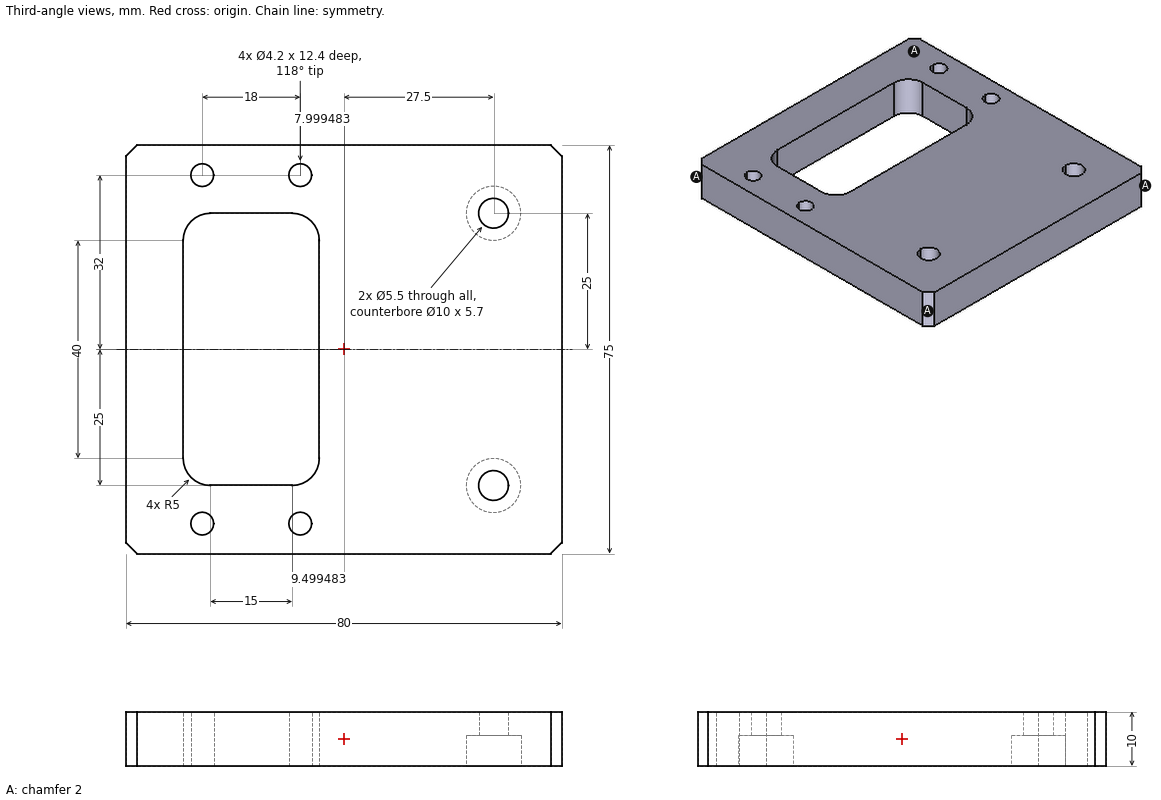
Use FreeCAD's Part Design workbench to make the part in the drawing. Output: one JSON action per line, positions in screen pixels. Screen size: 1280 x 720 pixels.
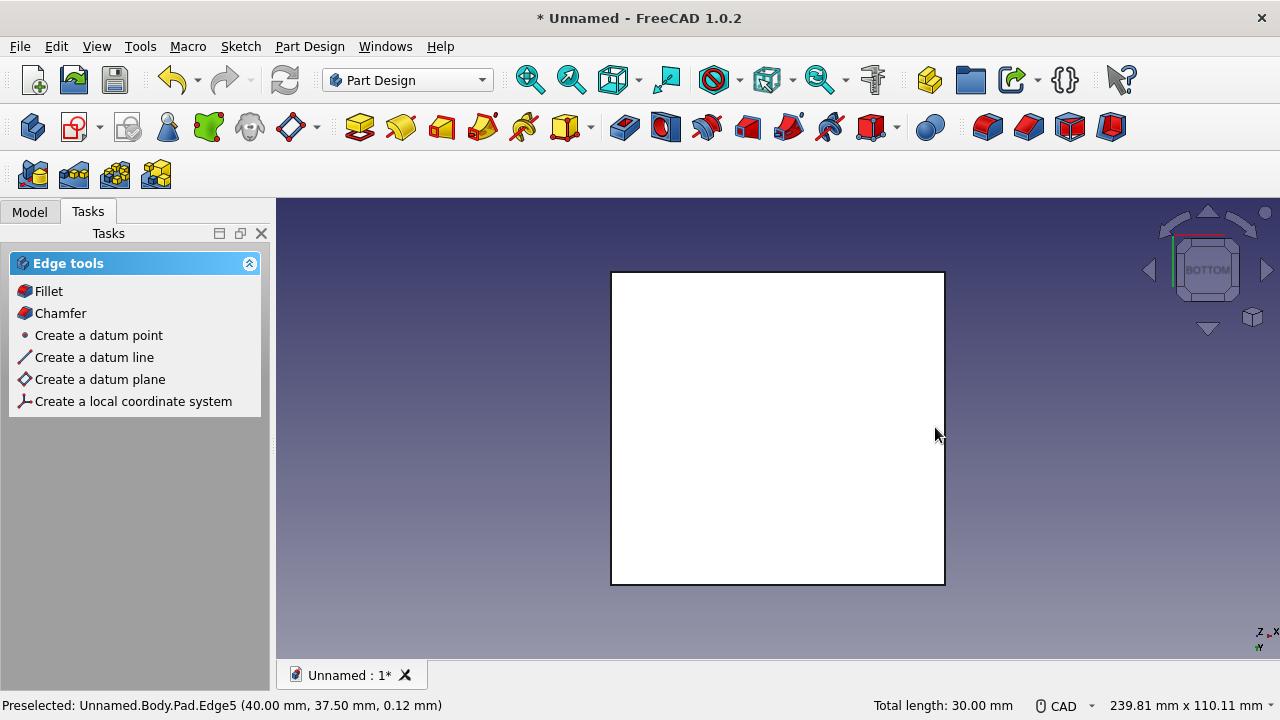
{"action": "key", "text": "4"}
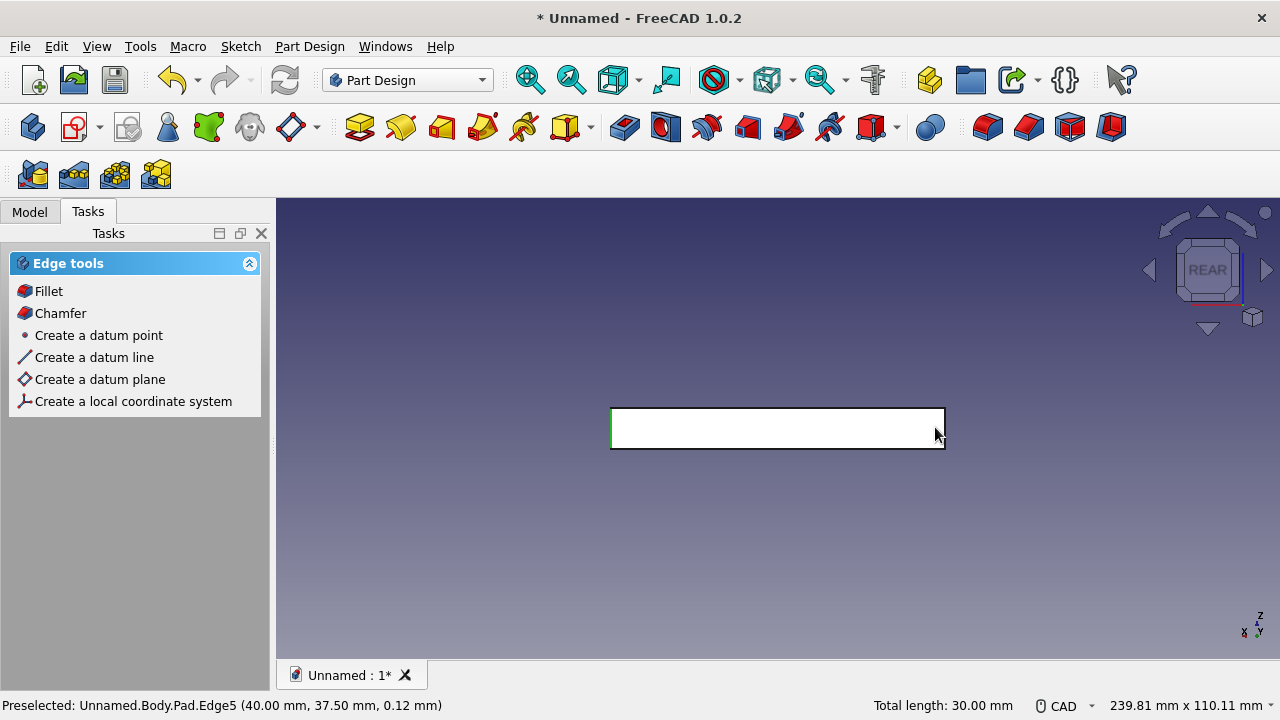
{"action": "key", "text": "v f"}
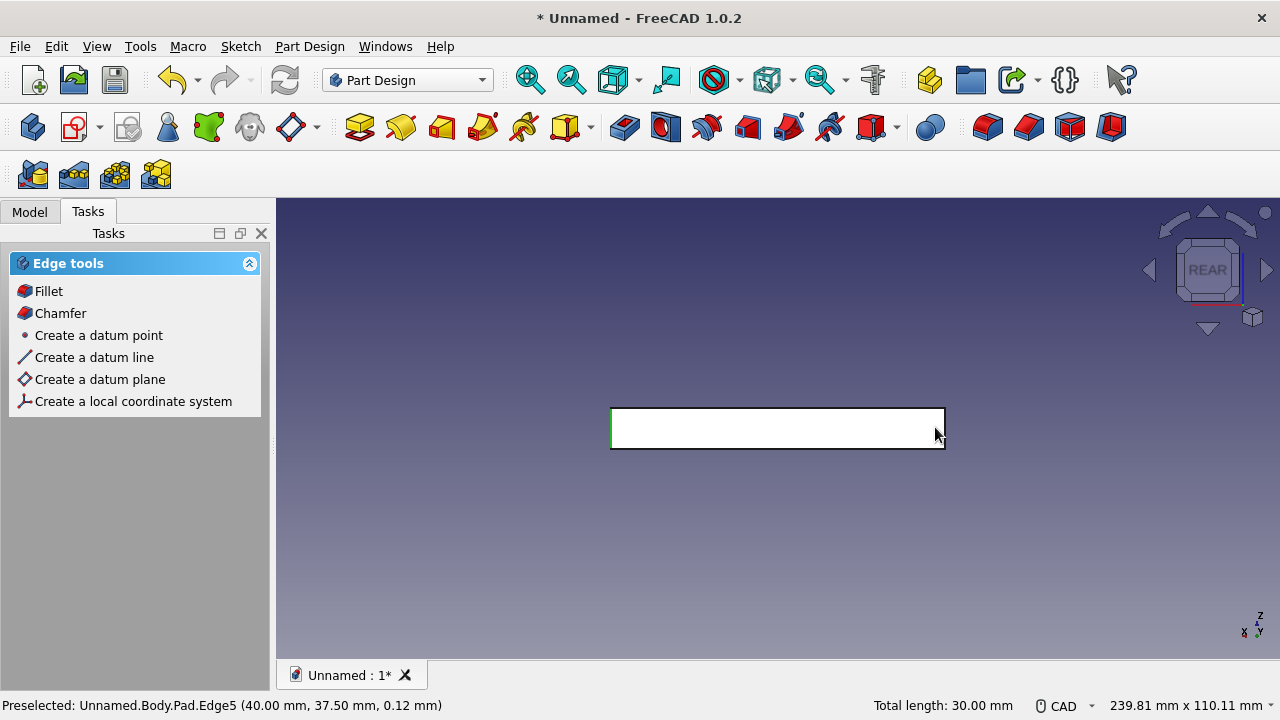
{"action": "left_click", "coordinate": [945, 428], "text": "ctrl"}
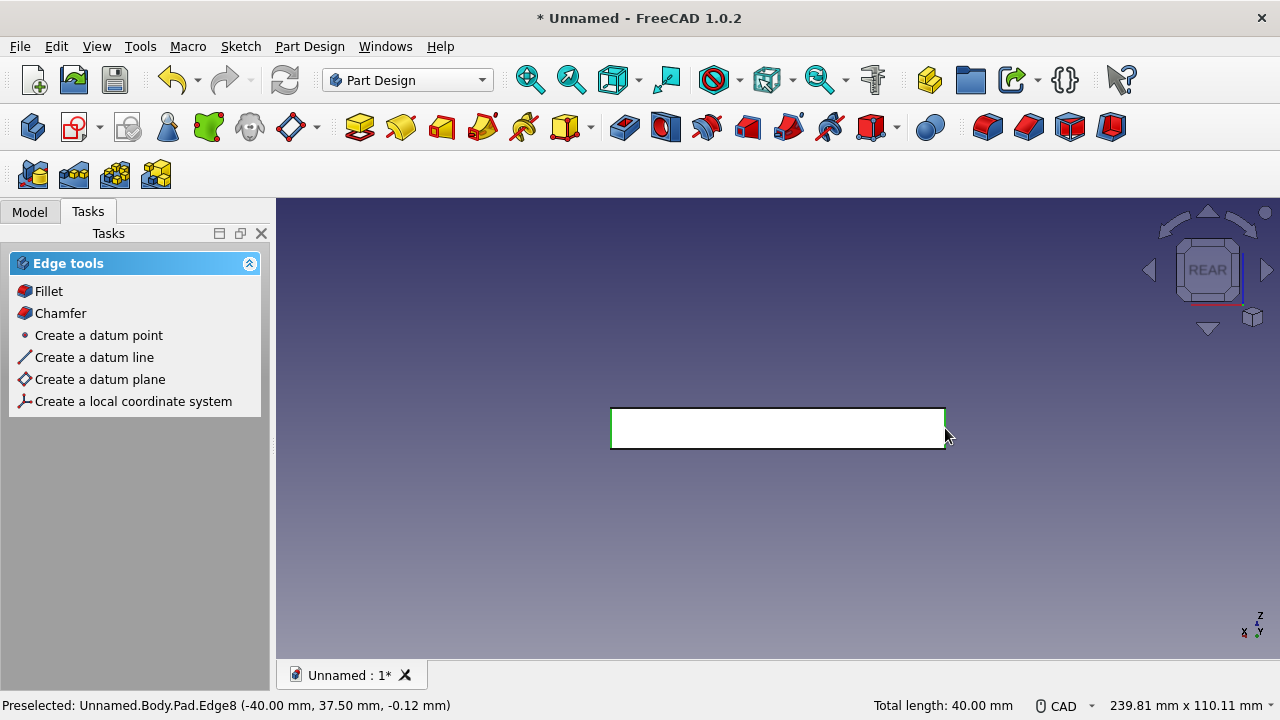
{"action": "left_click", "coordinate": [1029, 128]}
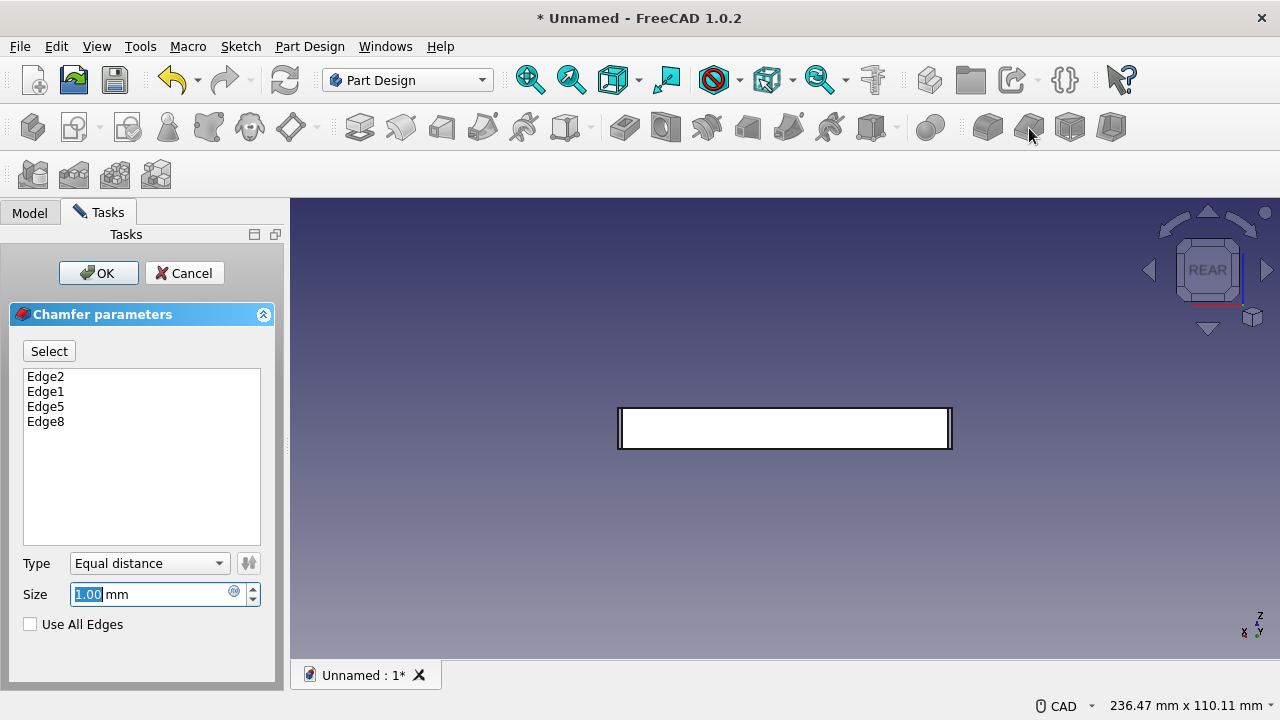
{"action": "type", "text": "2"}
{"action": "key", "text": "Tab"}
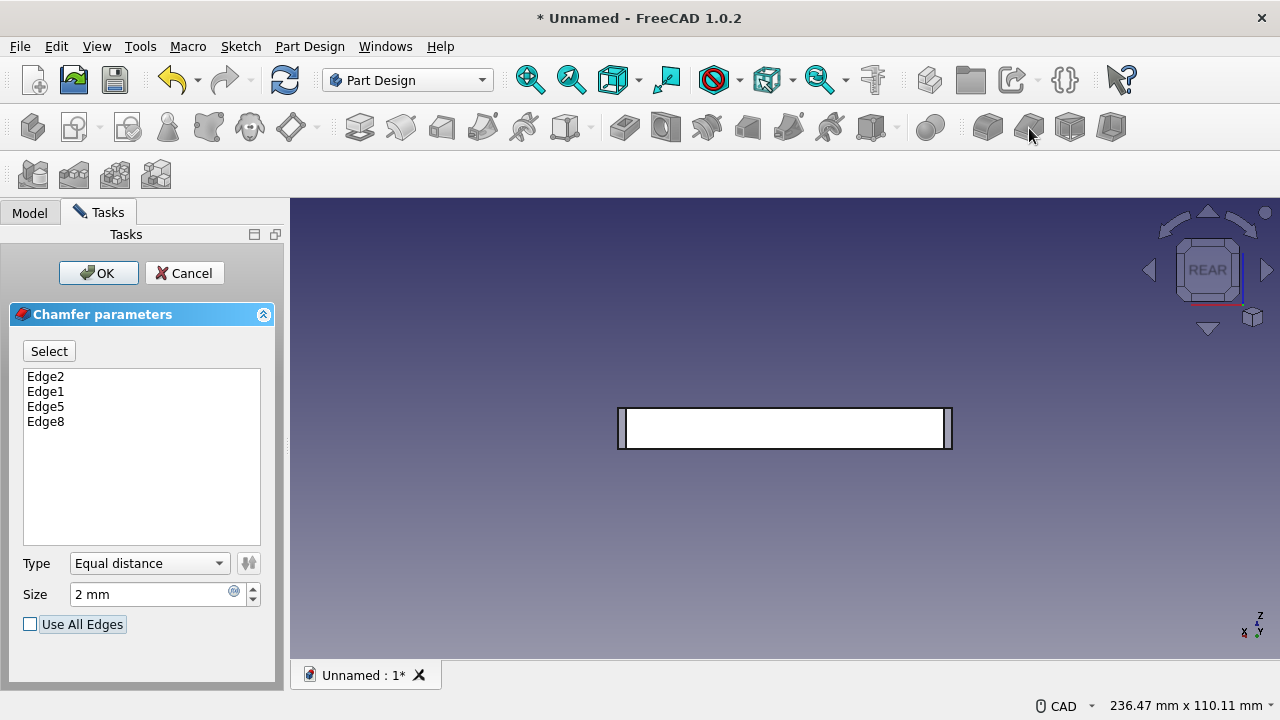
{"action": "left_click", "coordinate": [99, 273]}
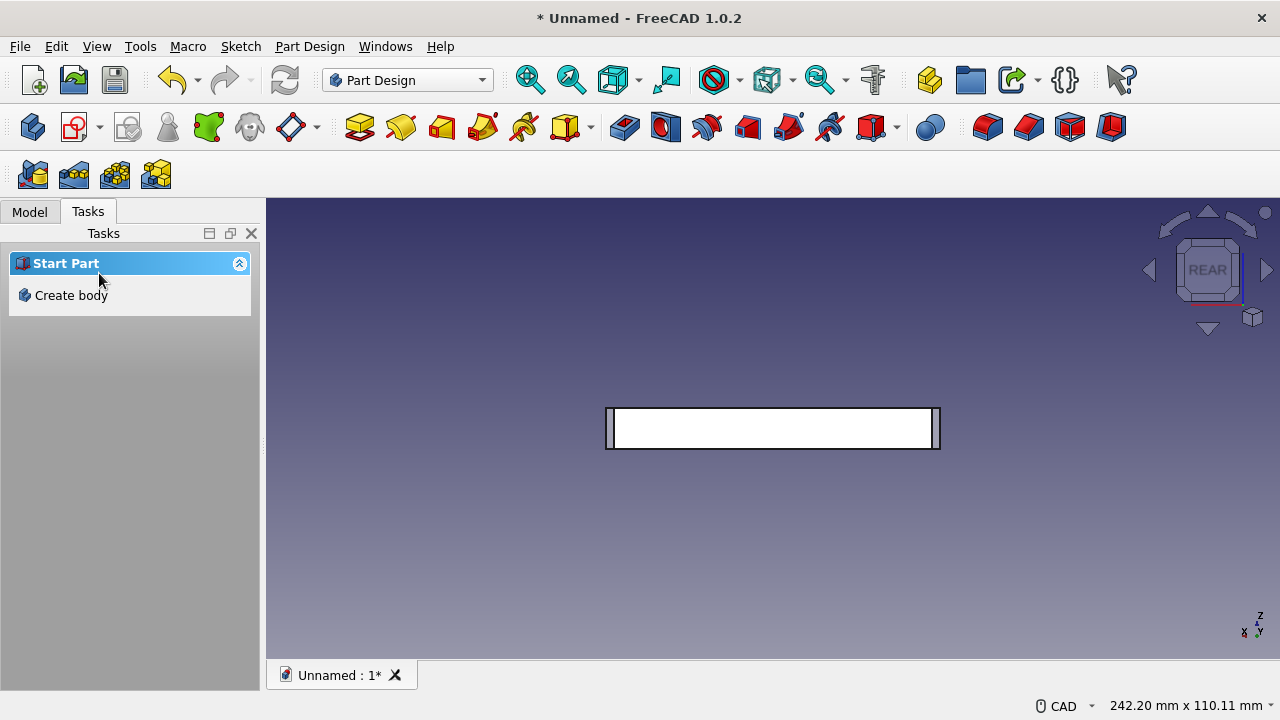
{"action": "key", "text": "v f"}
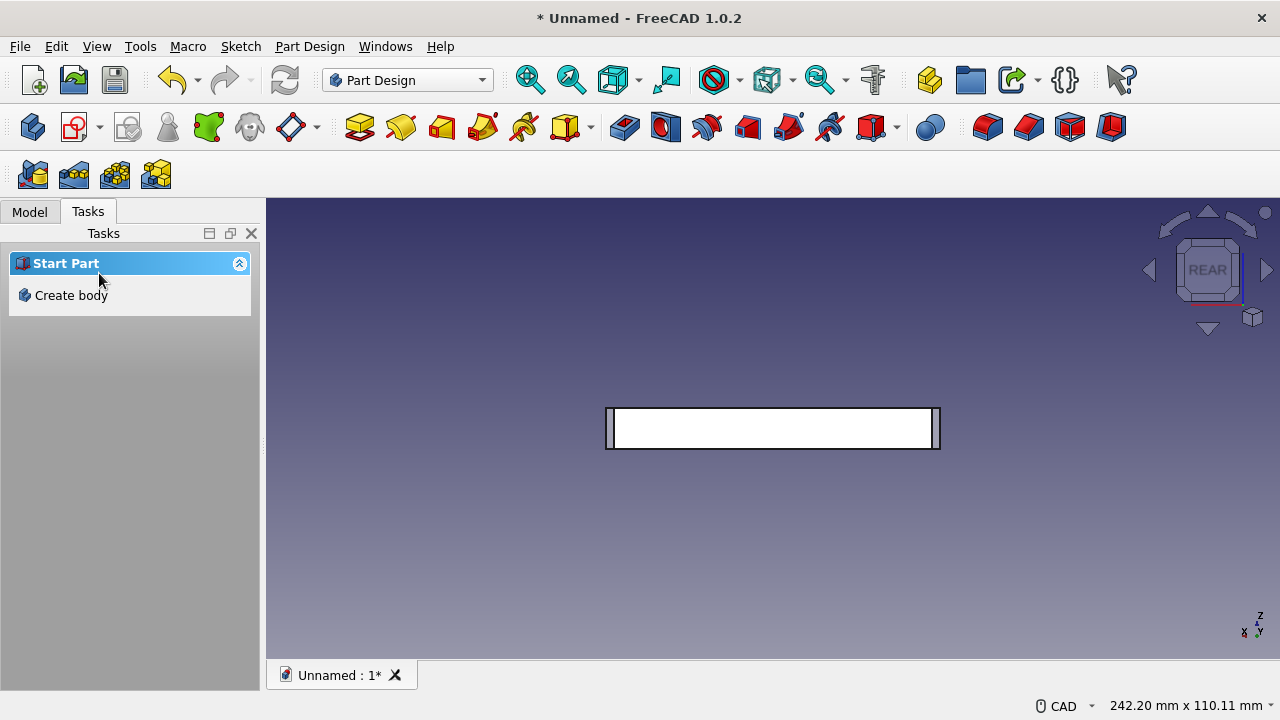
{"action": "key", "text": "5"}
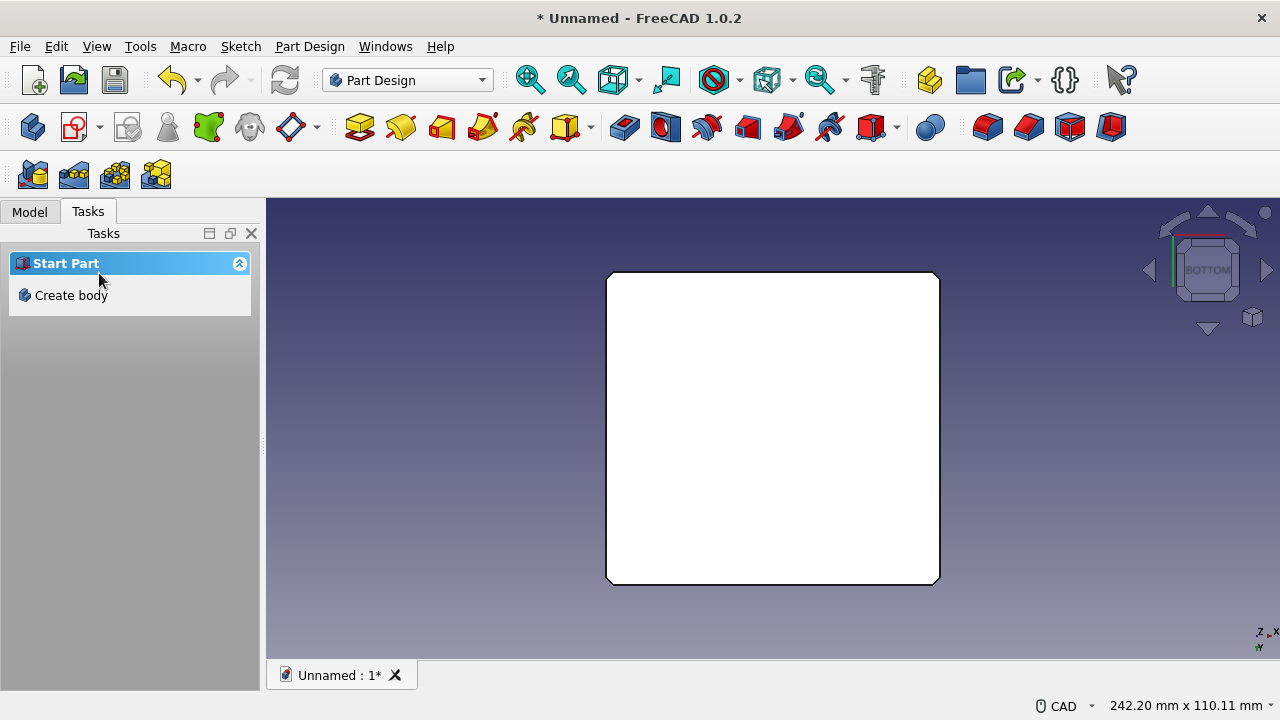
{"action": "left_click", "coordinate": [773, 427]}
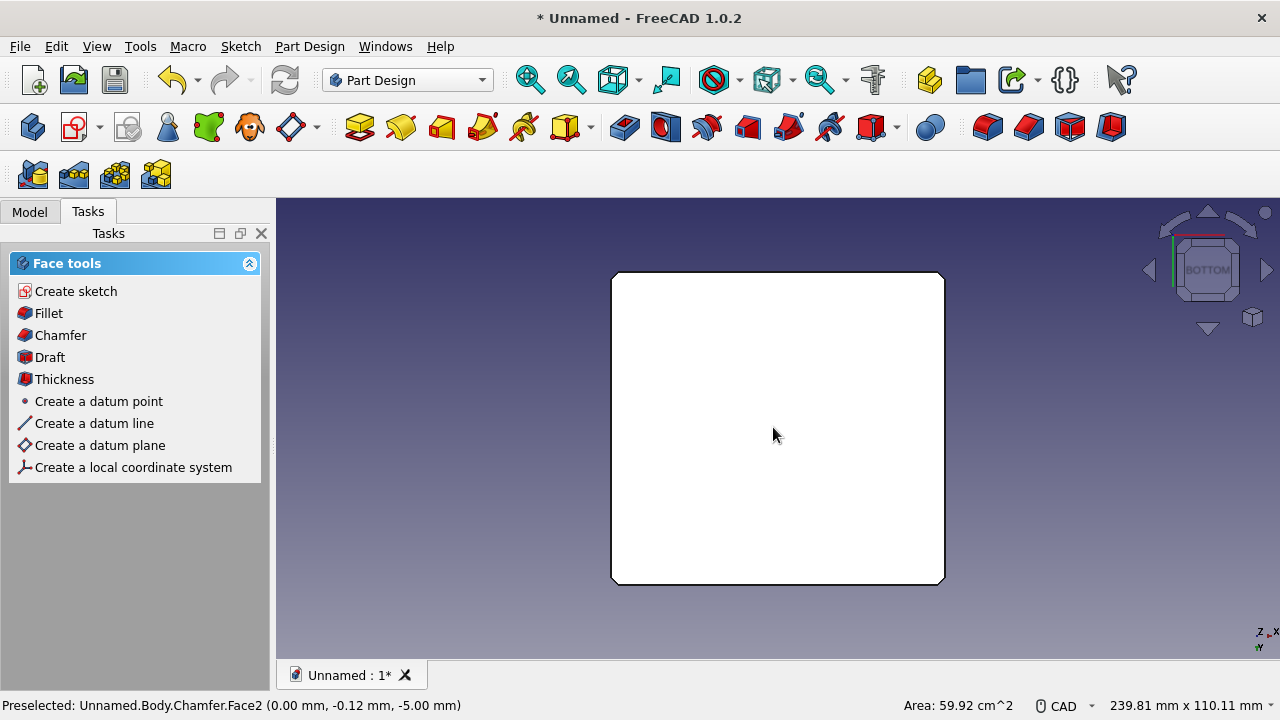
{"action": "left_click", "coordinate": [74, 128]}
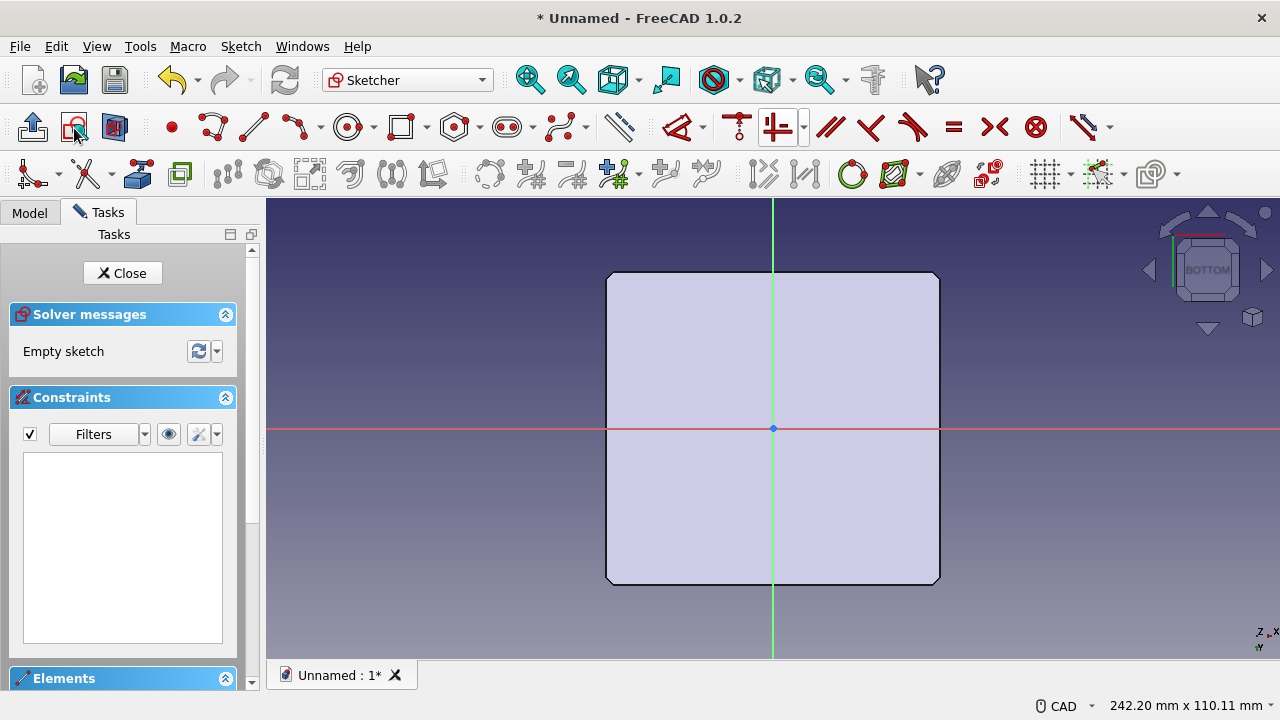
{"action": "key", "text": "g c"}